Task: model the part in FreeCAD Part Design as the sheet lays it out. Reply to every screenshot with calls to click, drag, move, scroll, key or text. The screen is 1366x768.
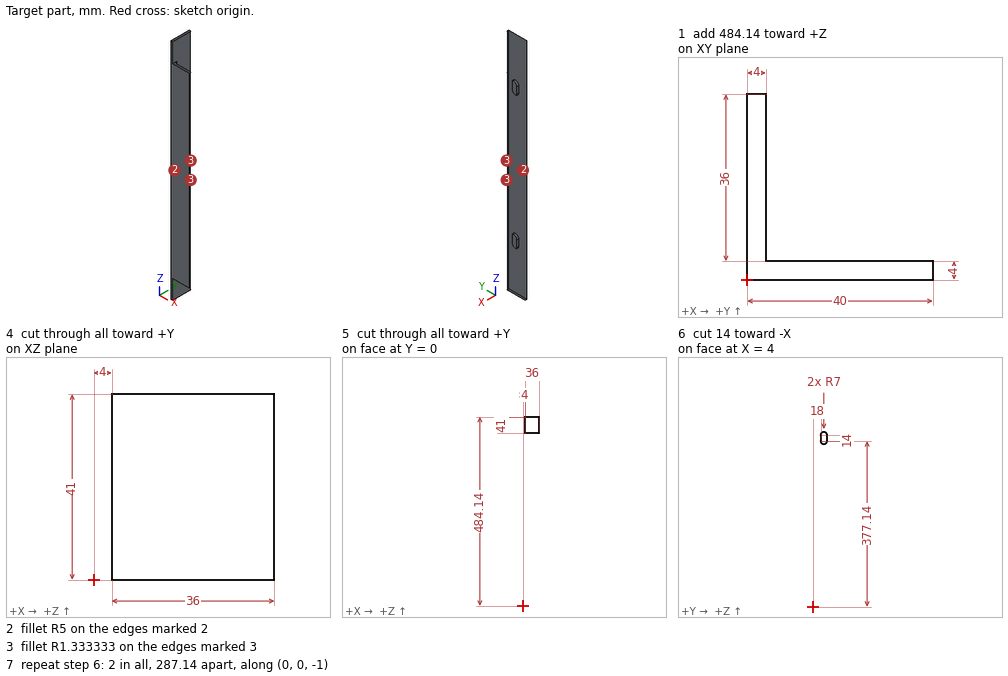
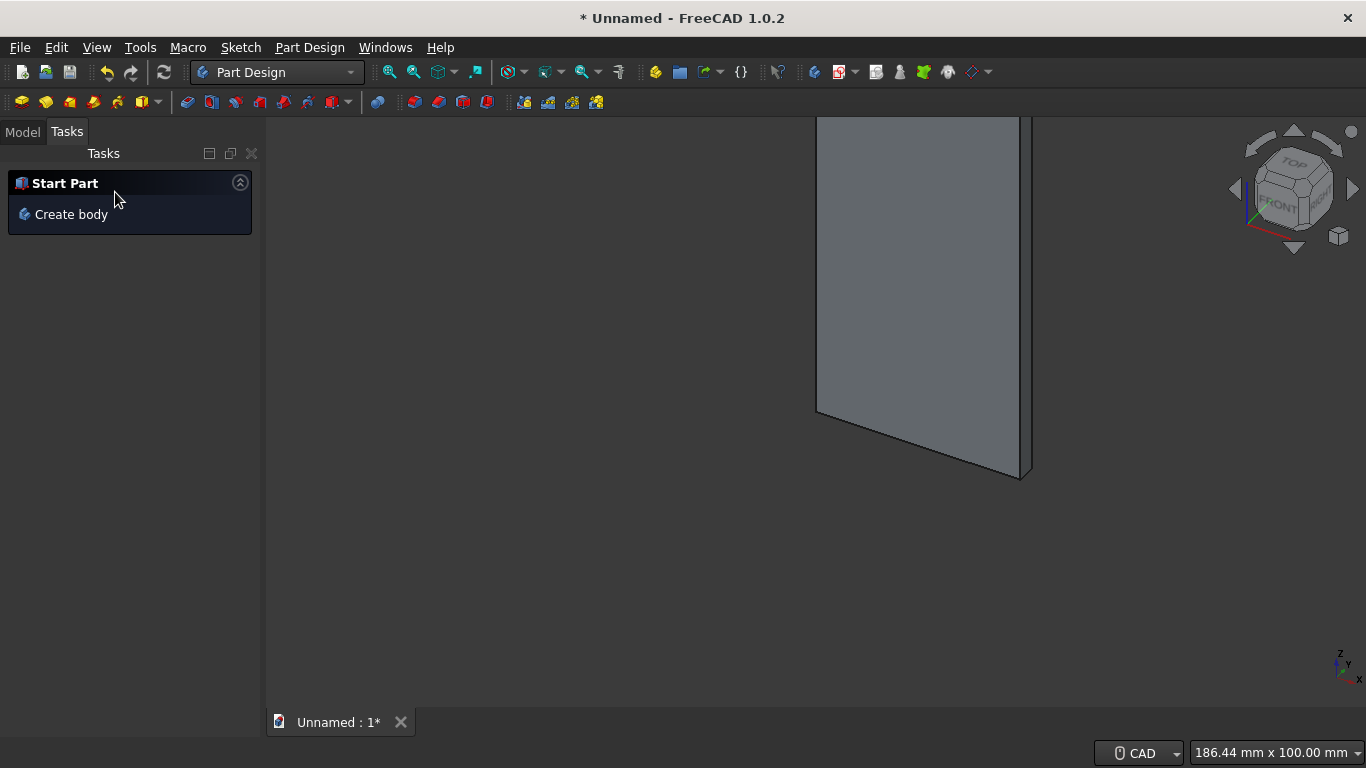
click(390, 72)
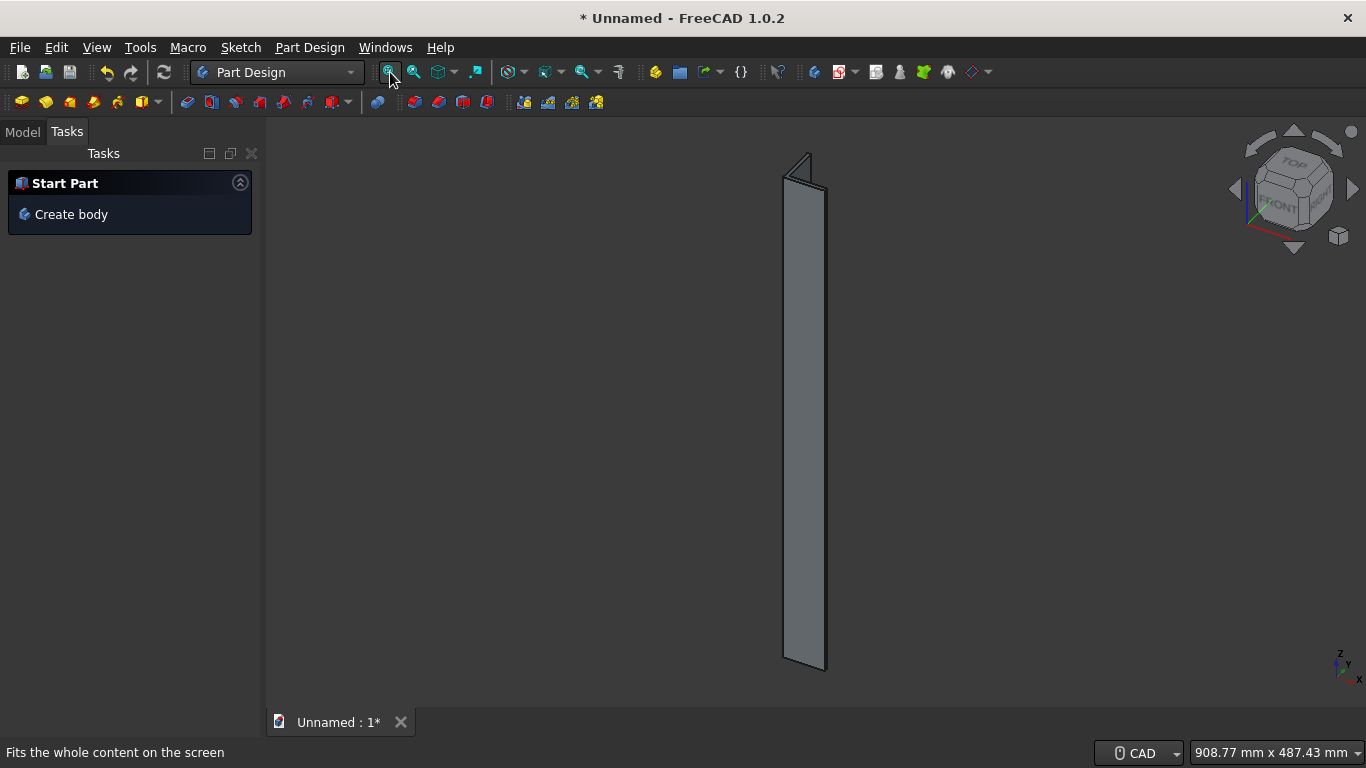
key(0)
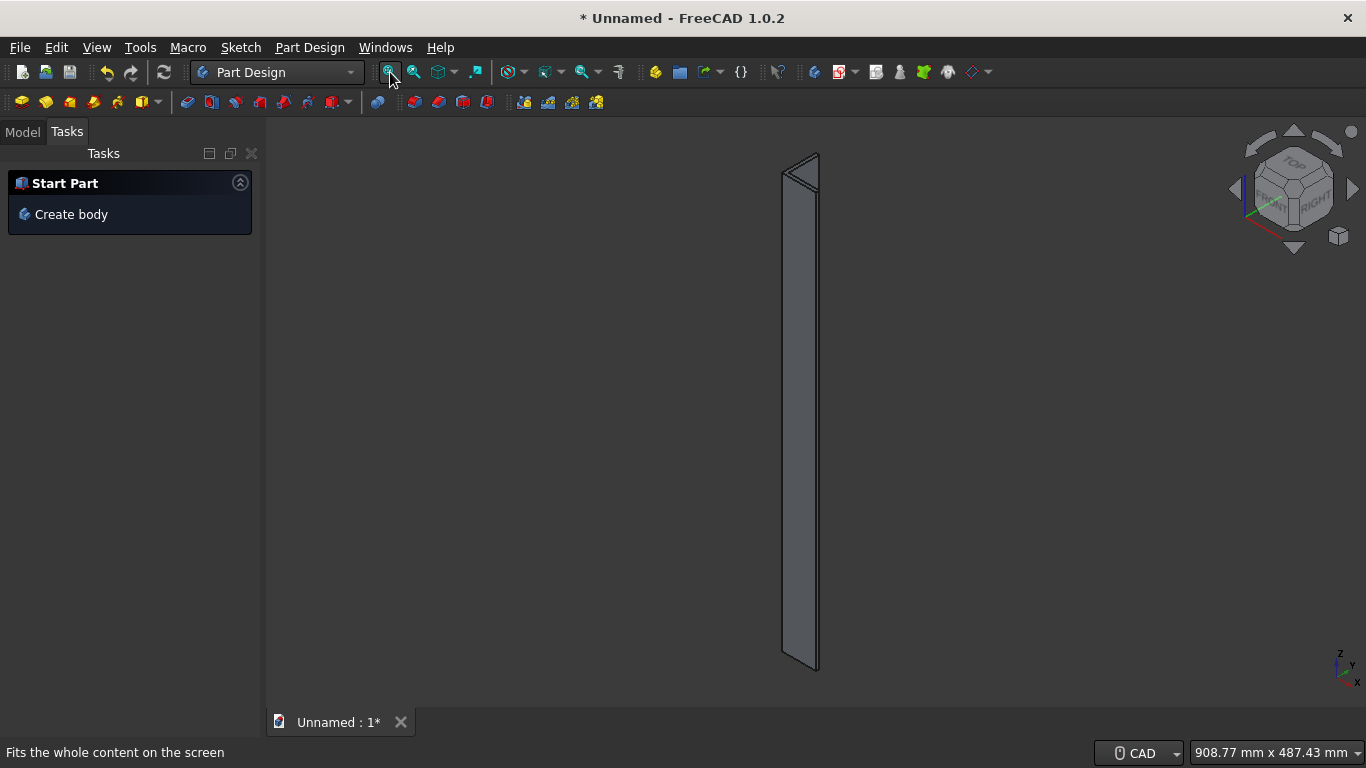
key(2)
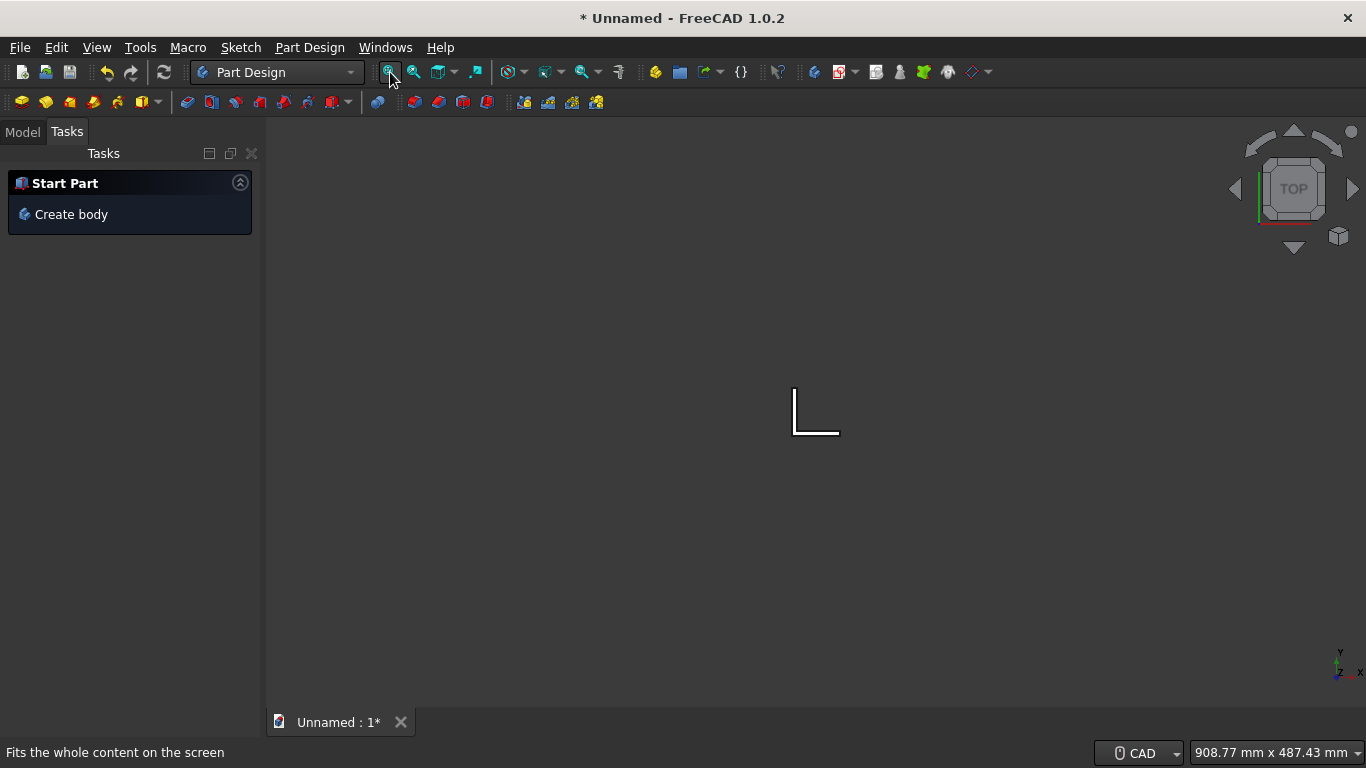
click(390, 72)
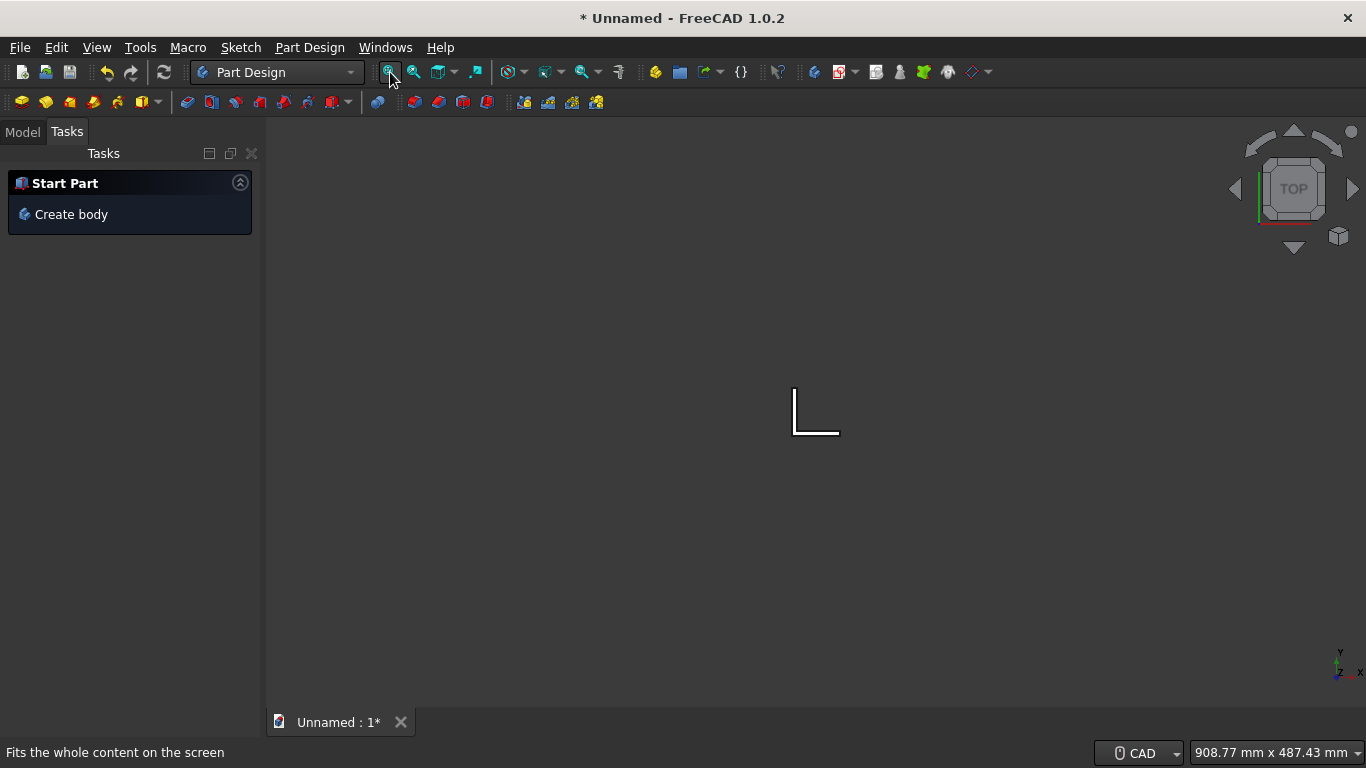
key(1)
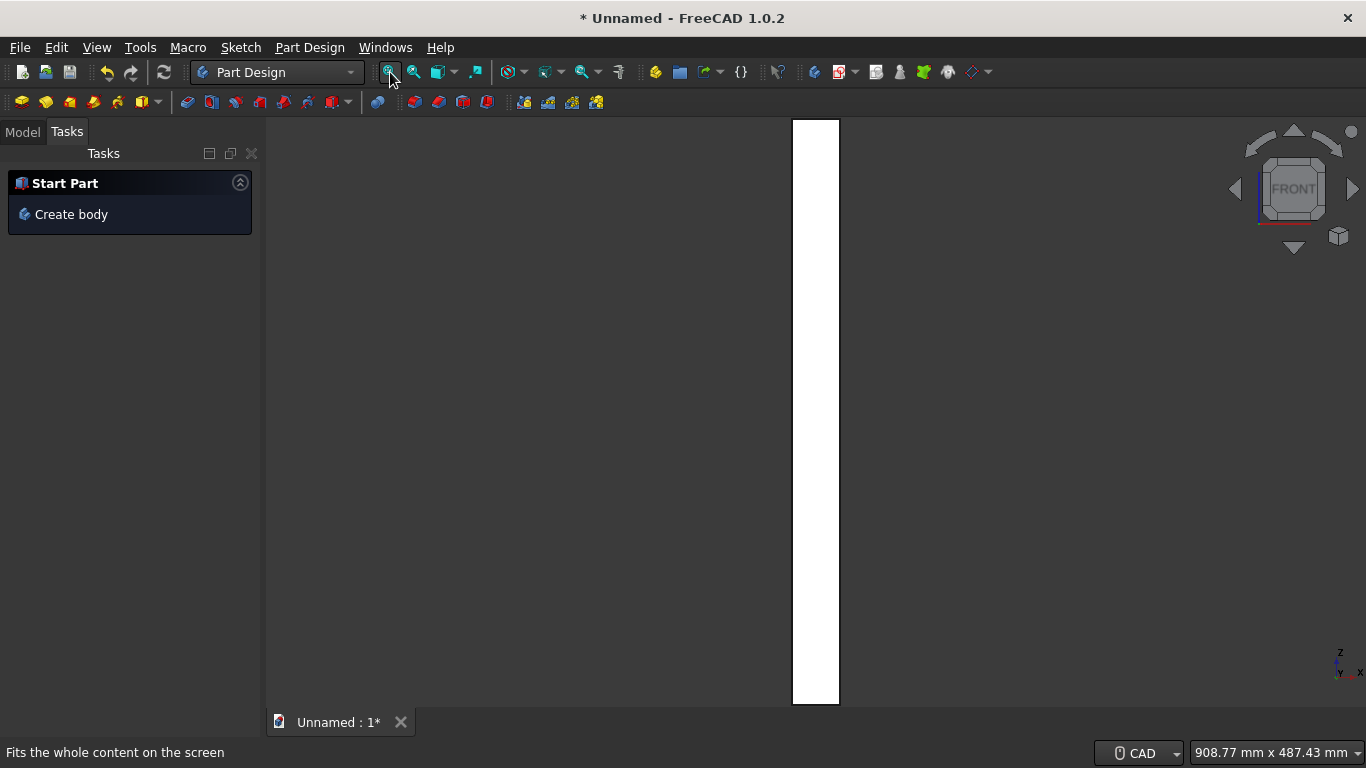
key(3)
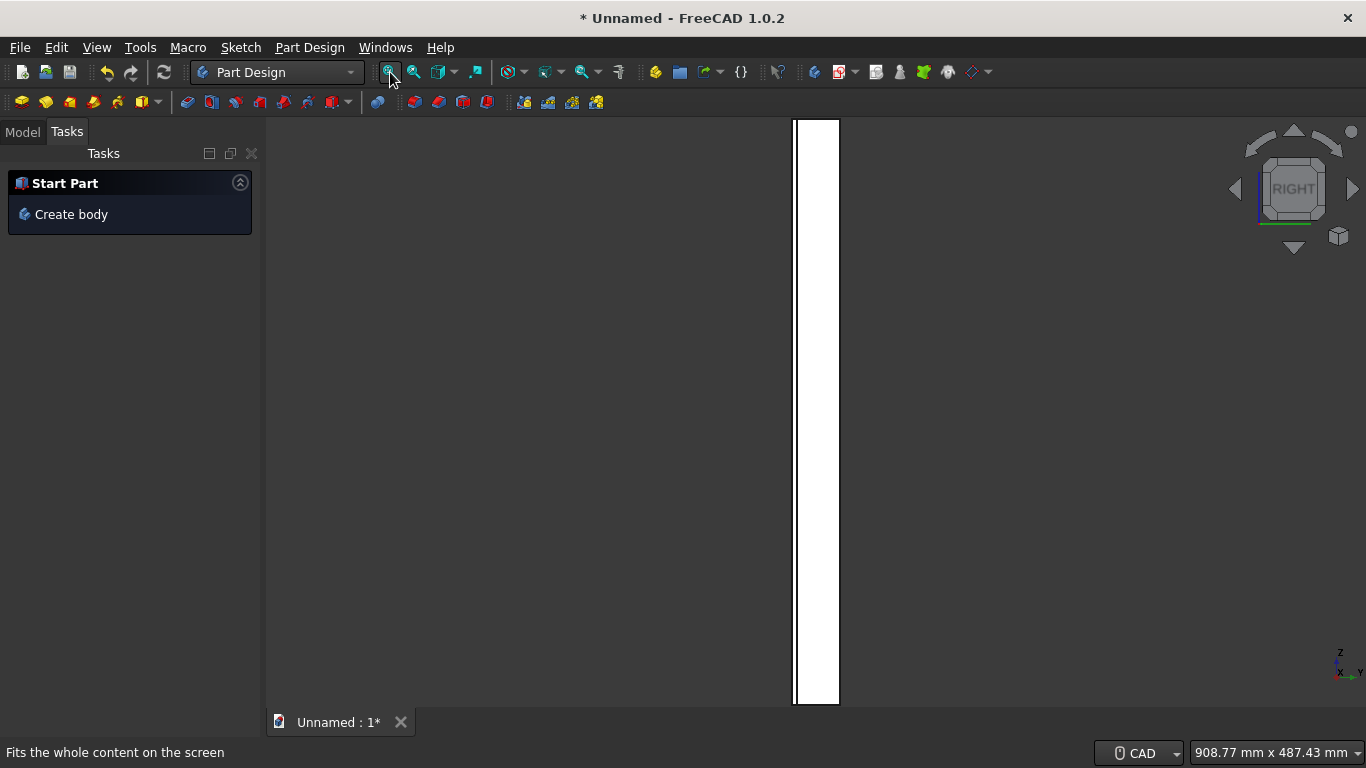
key(5)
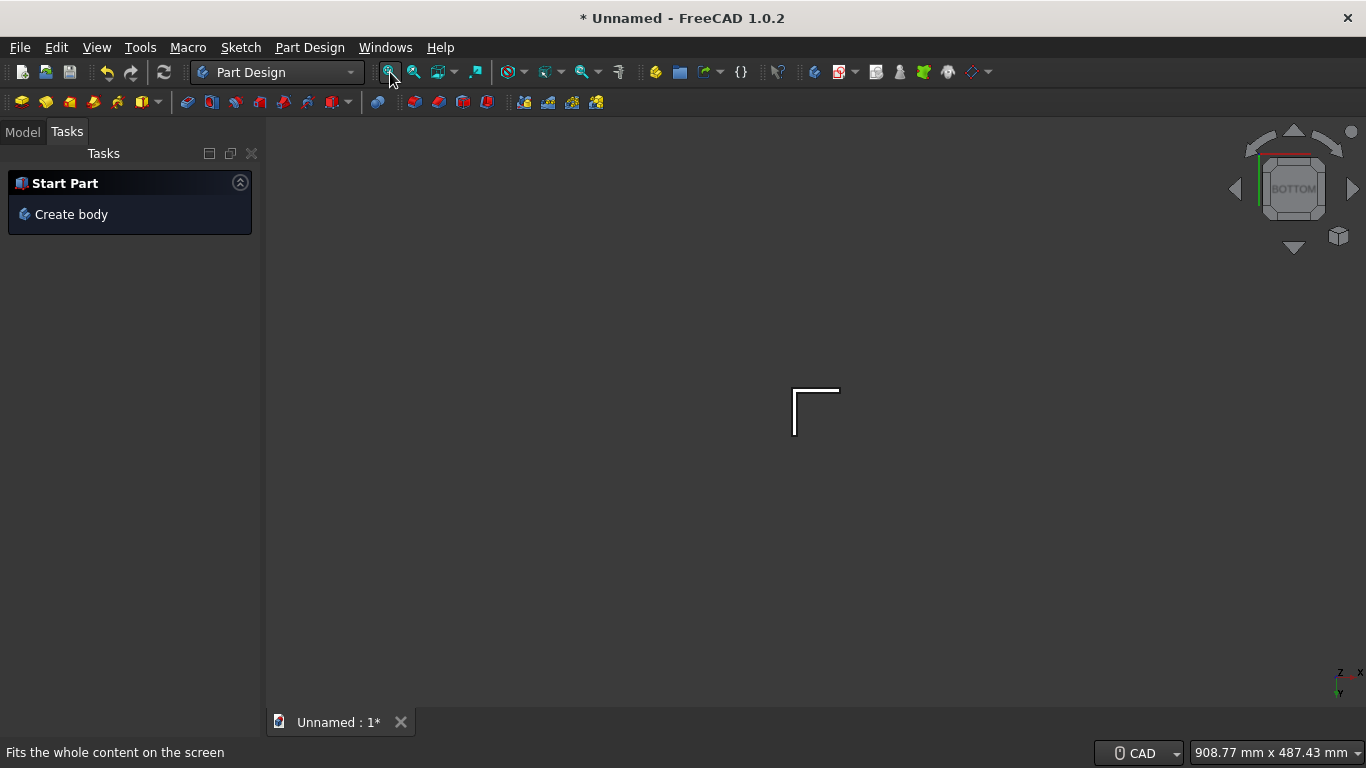
click(390, 72)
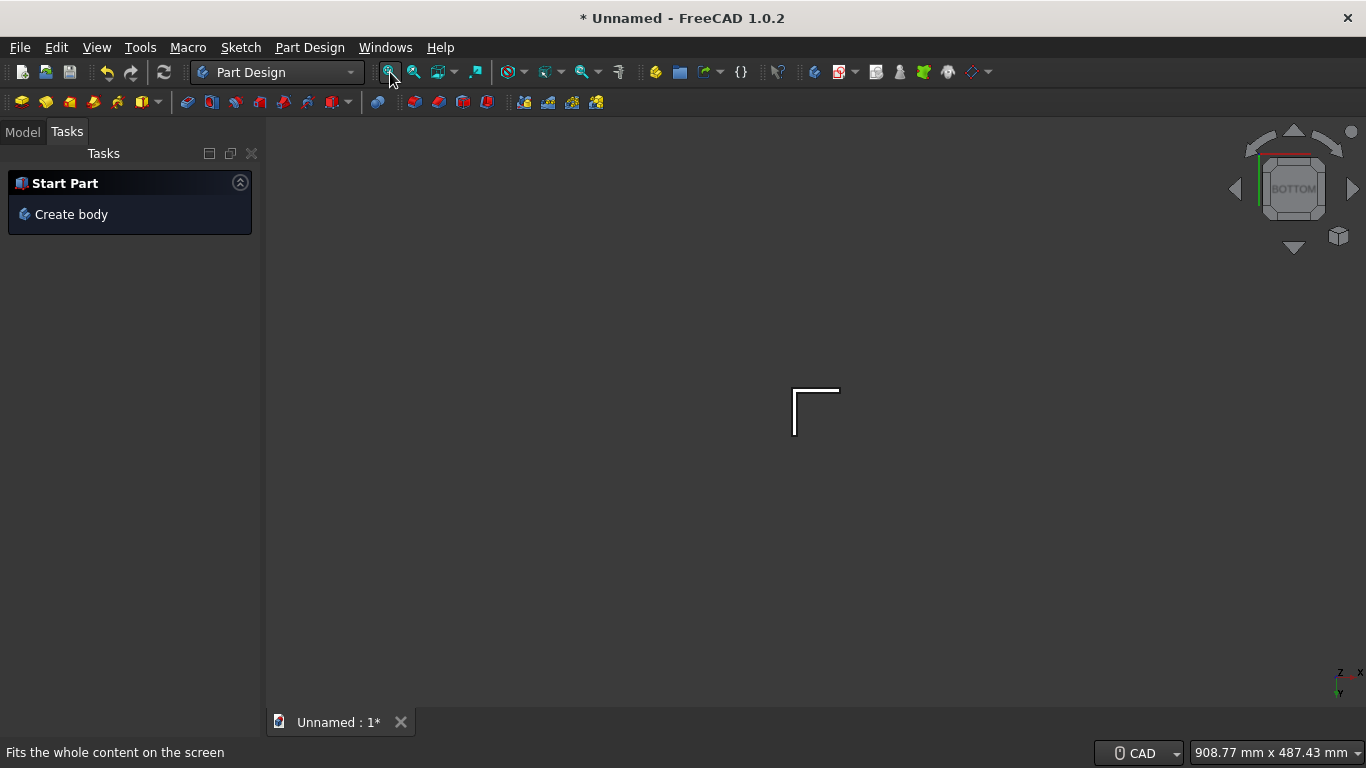
key(4)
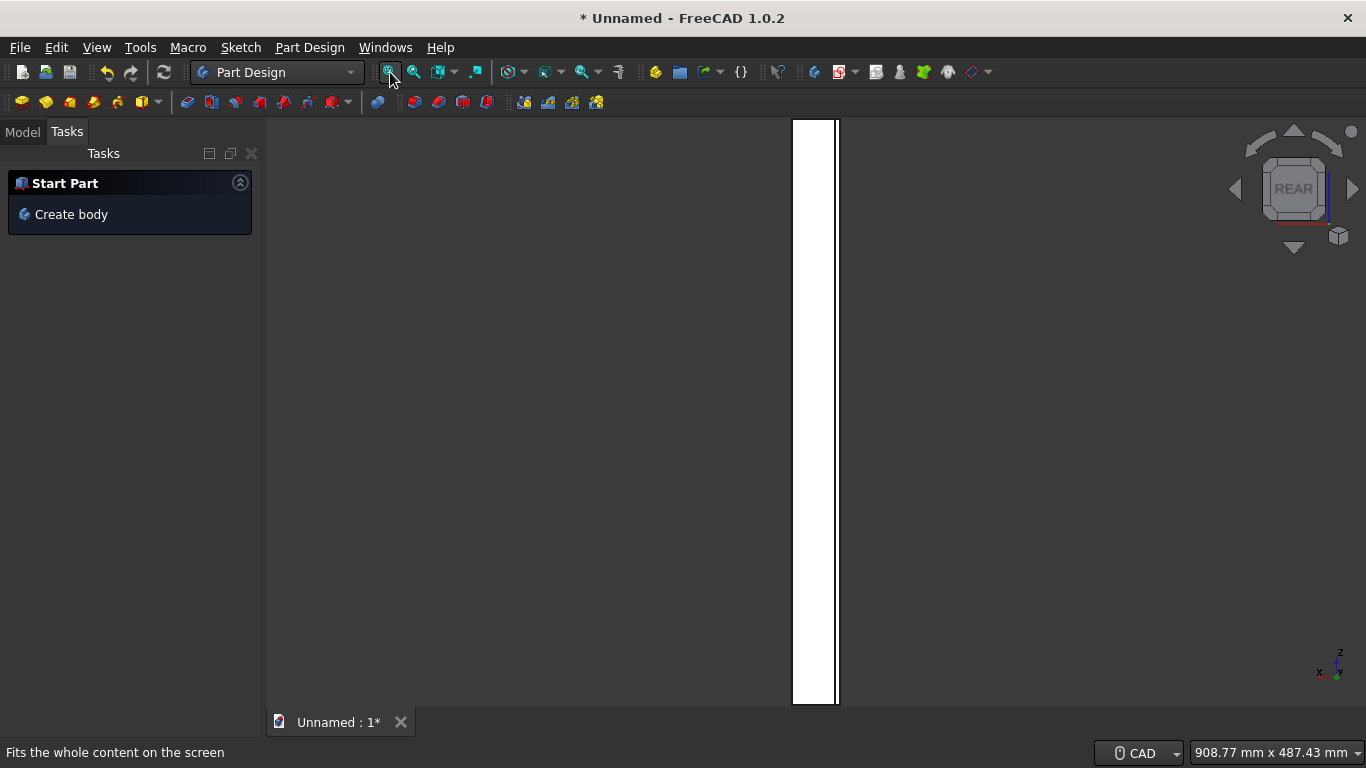
key(6)